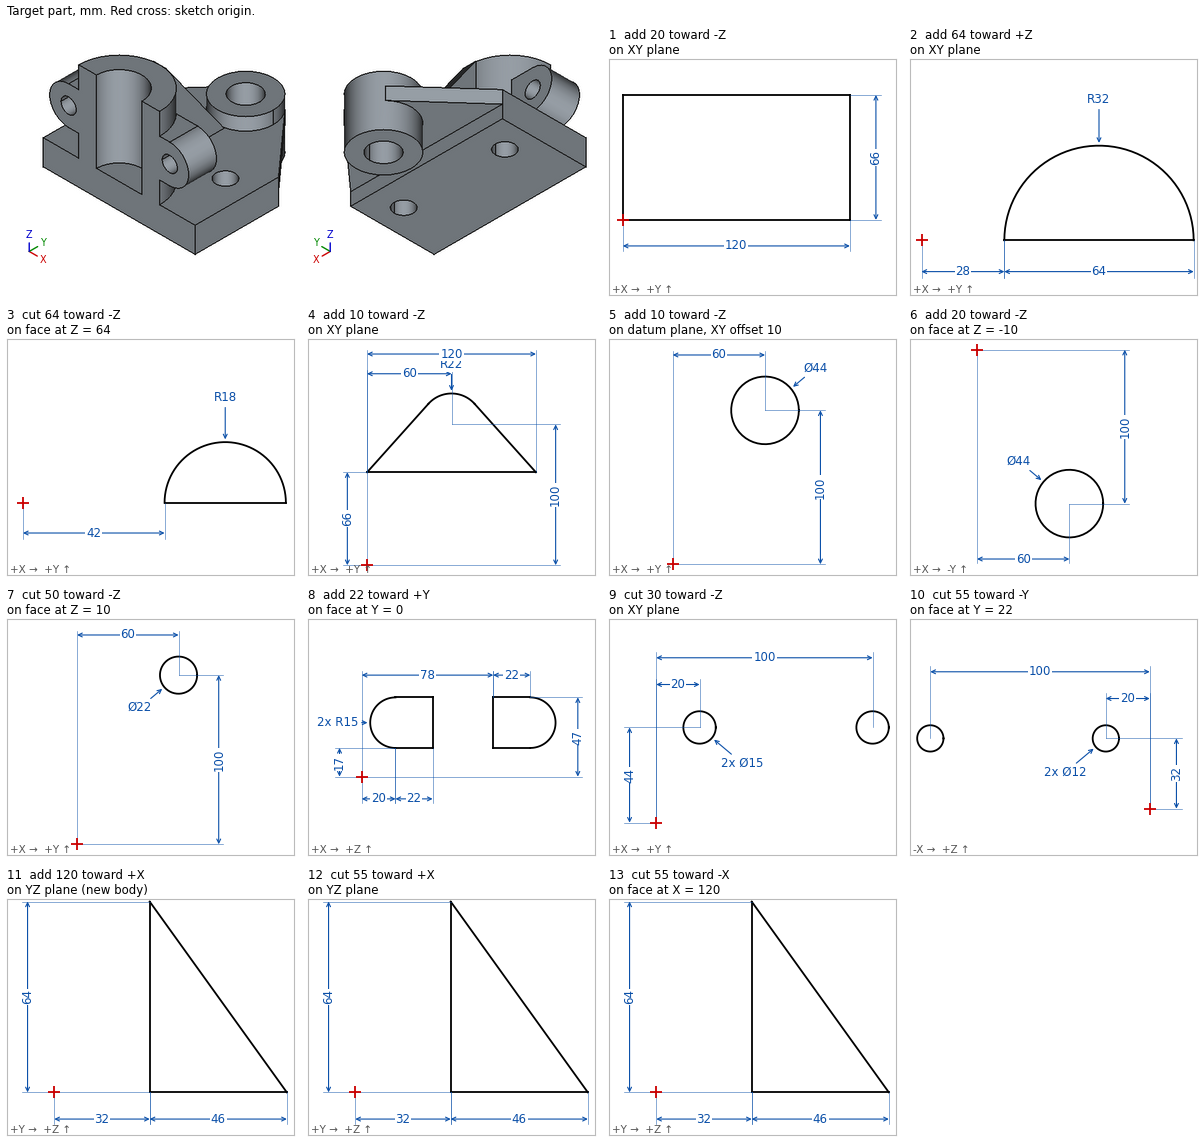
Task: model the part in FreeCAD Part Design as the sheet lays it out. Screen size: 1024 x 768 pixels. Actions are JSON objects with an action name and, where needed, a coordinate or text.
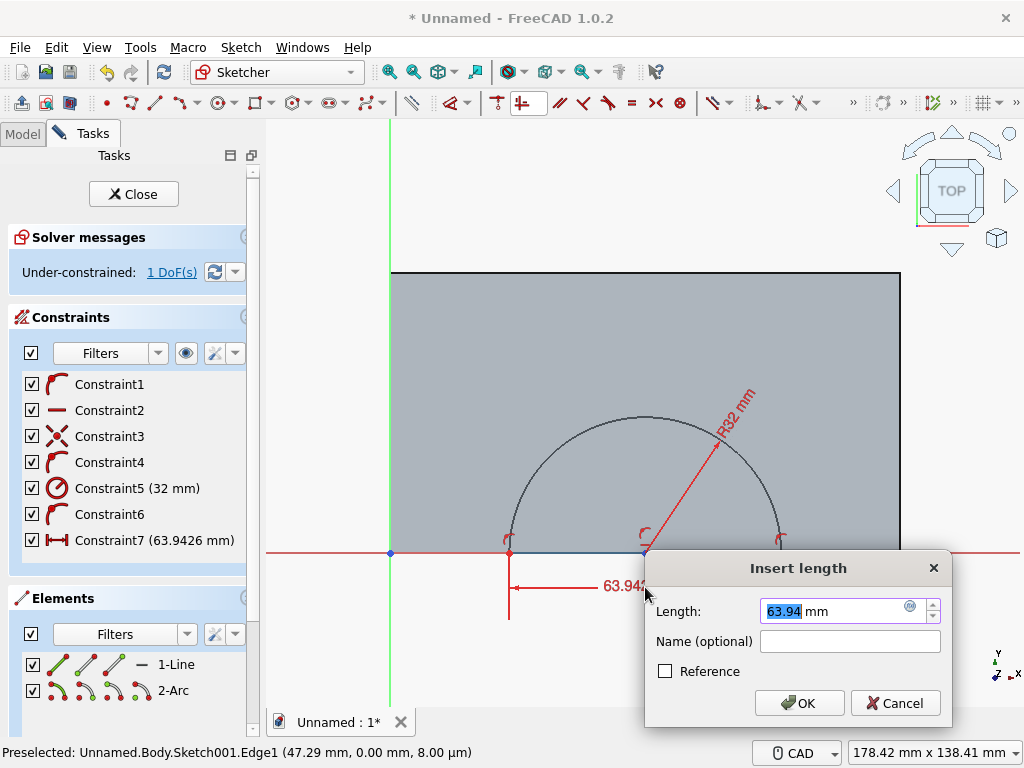
{"action": "type", "text": "64"}
{"action": "key", "text": "Return"}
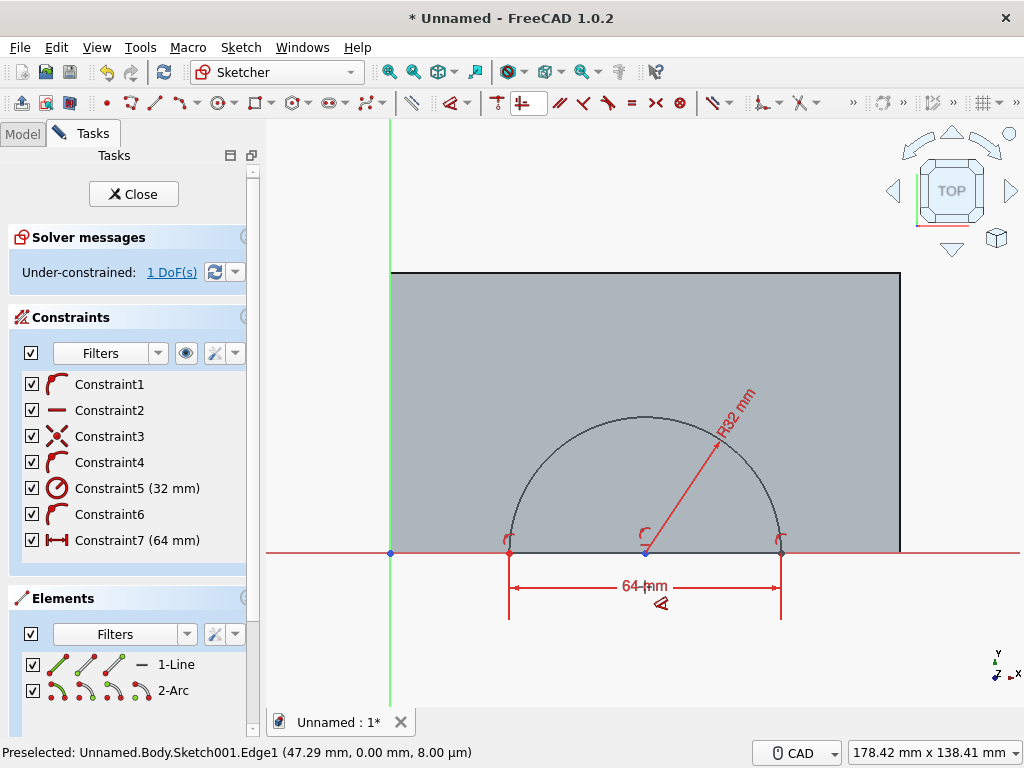
{"action": "left_click", "coordinate": [509, 553]}
{"action": "left_click", "coordinate": [450, 587]}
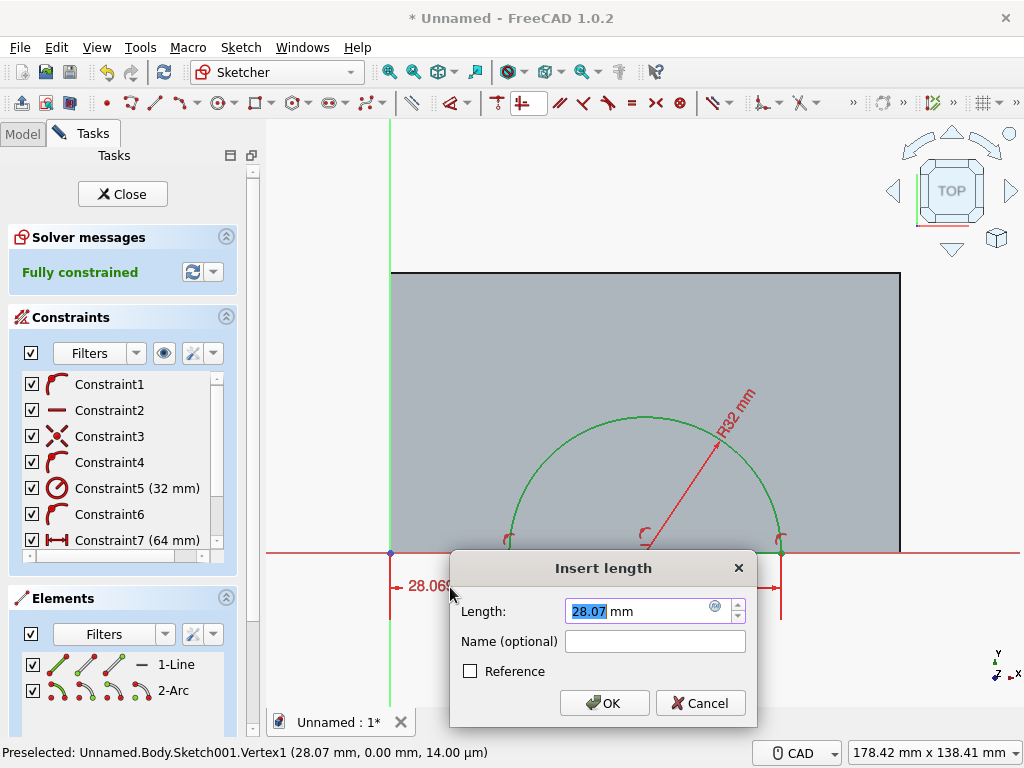
{"action": "type", "text": "28"}
{"action": "key", "text": "Return"}
{"action": "key", "text": "Escape"}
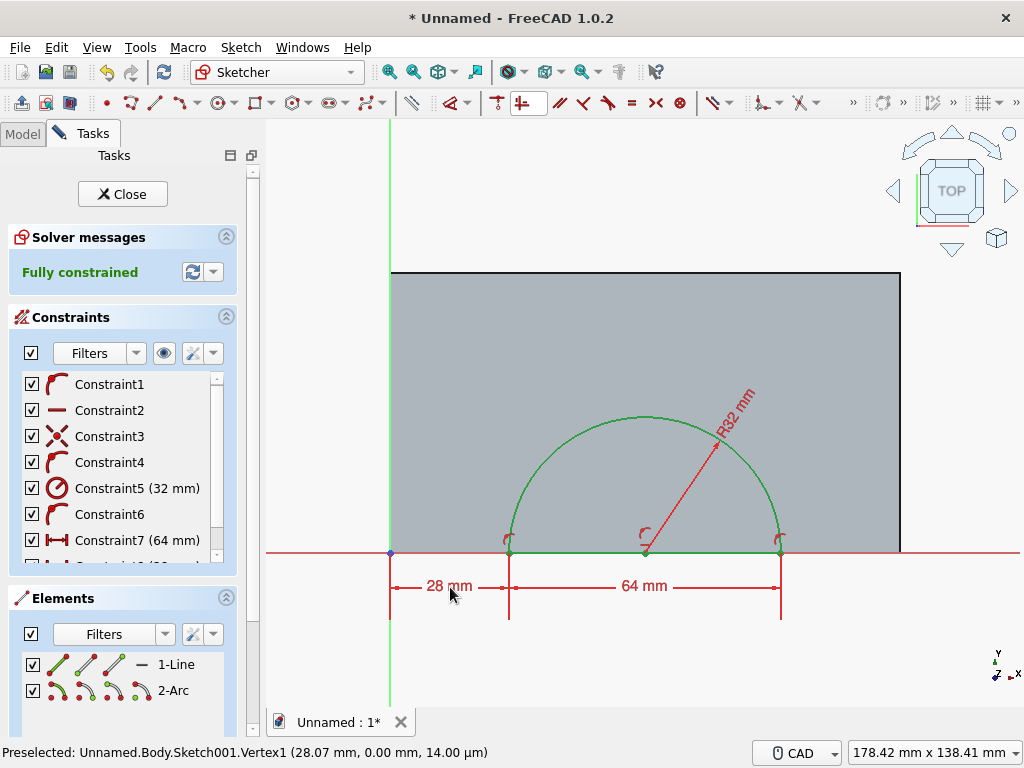
{"action": "left_click", "coordinate": [123, 194]}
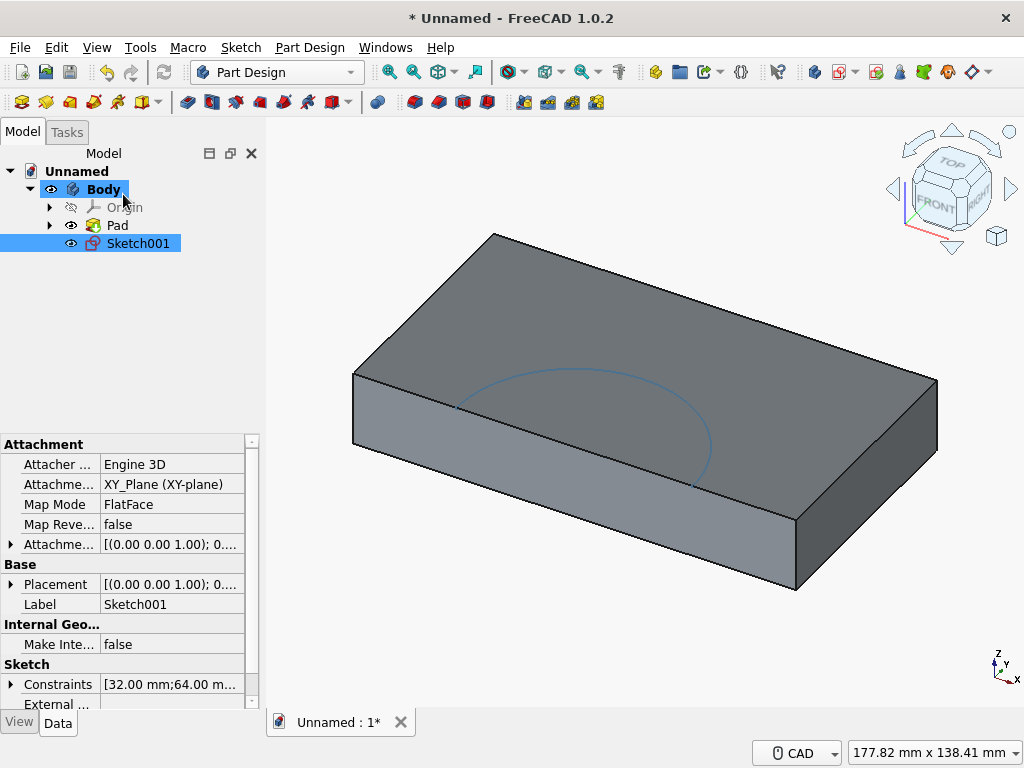
{"action": "left_click", "coordinate": [22, 102]}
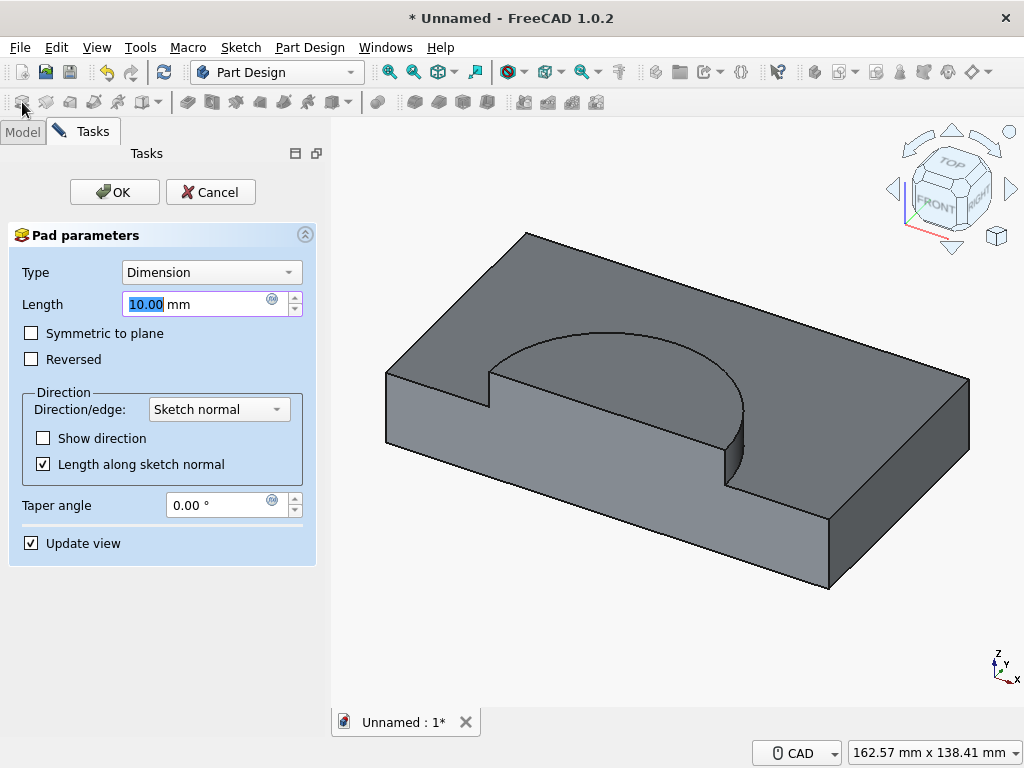
{"action": "type", "text": "64"}
{"action": "key", "text": "Tab"}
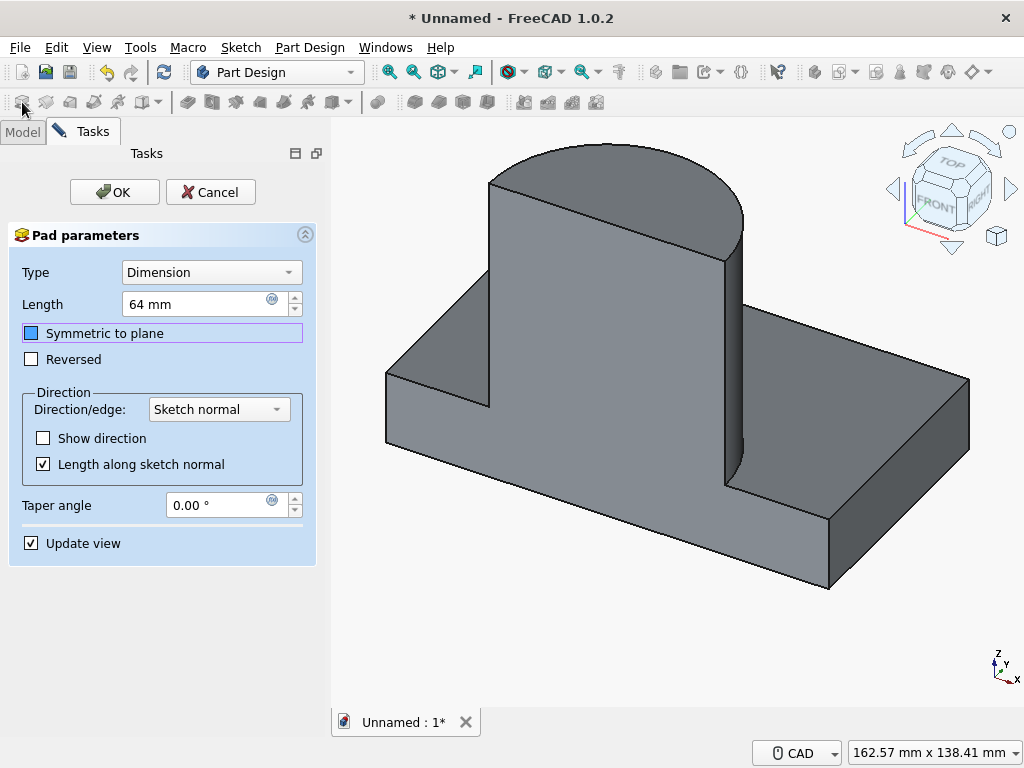
{"action": "left_click", "coordinate": [115, 192]}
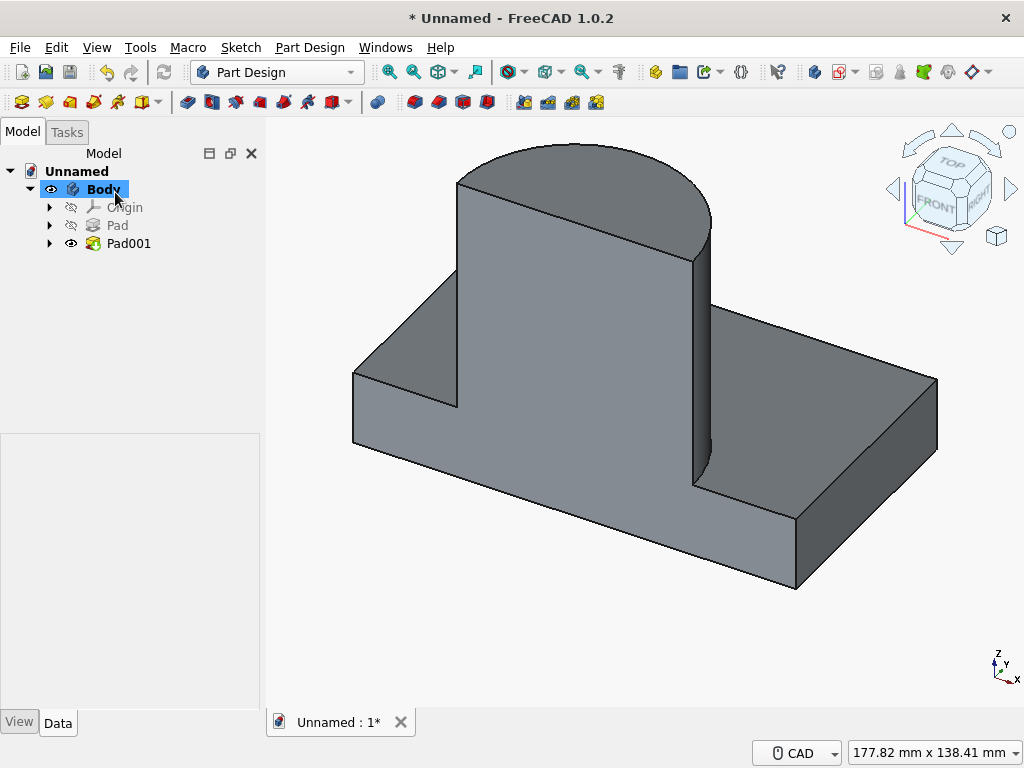
{"action": "left_click", "coordinate": [390, 72]}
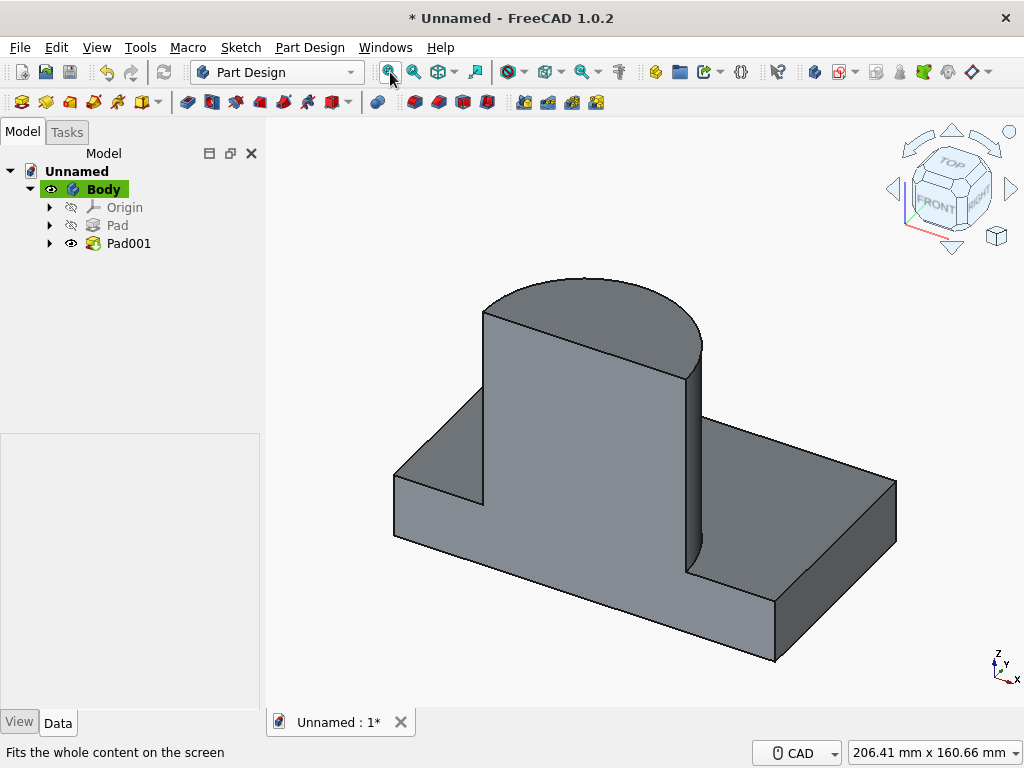
{"action": "left_click", "coordinate": [614, 316]}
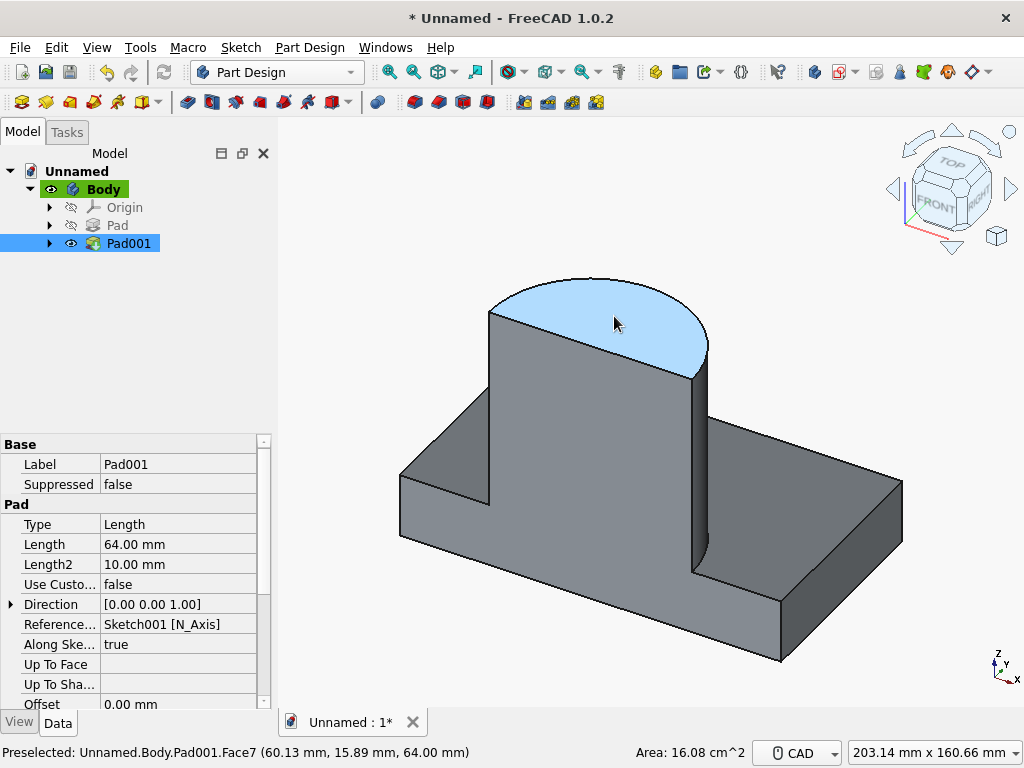
{"action": "left_click", "coordinate": [840, 72]}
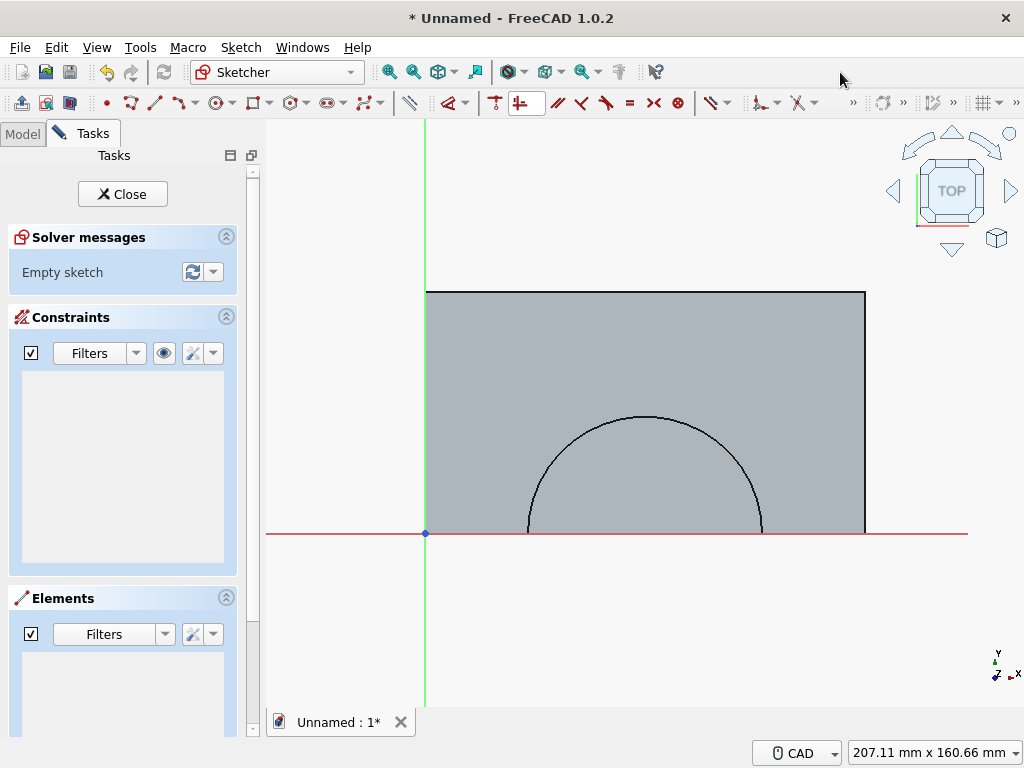
{"action": "scroll", "coordinate": [551, 679], "scroll_direction": "up", "scroll_amount": 2}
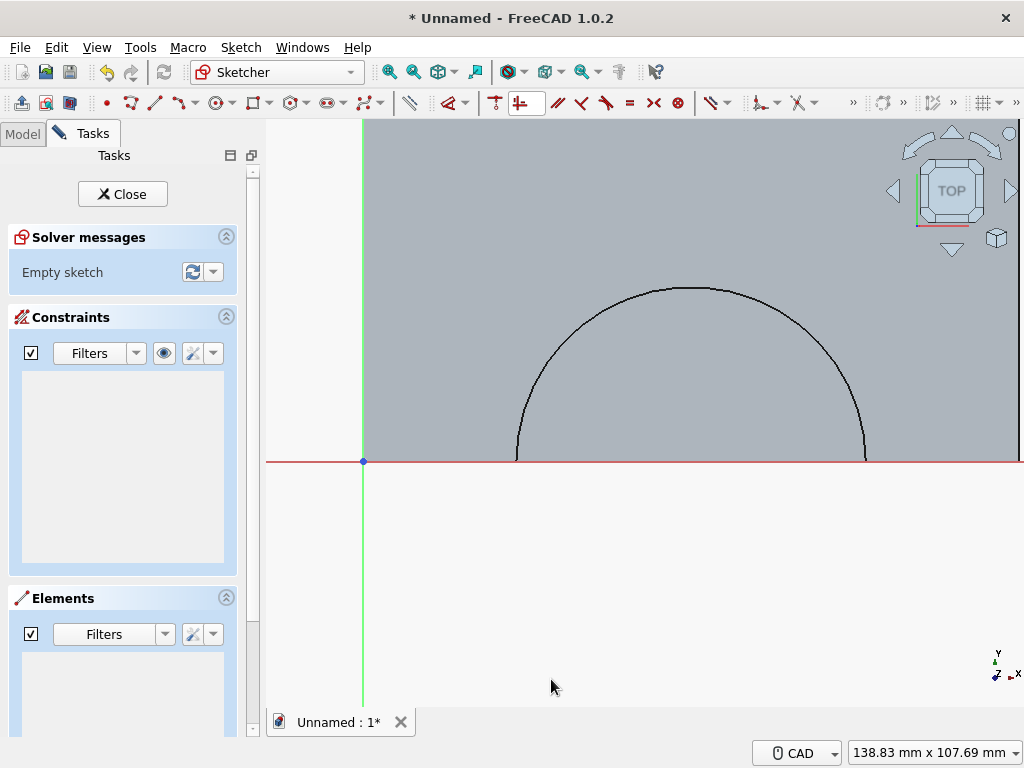
{"action": "left_click", "coordinate": [156, 104]}